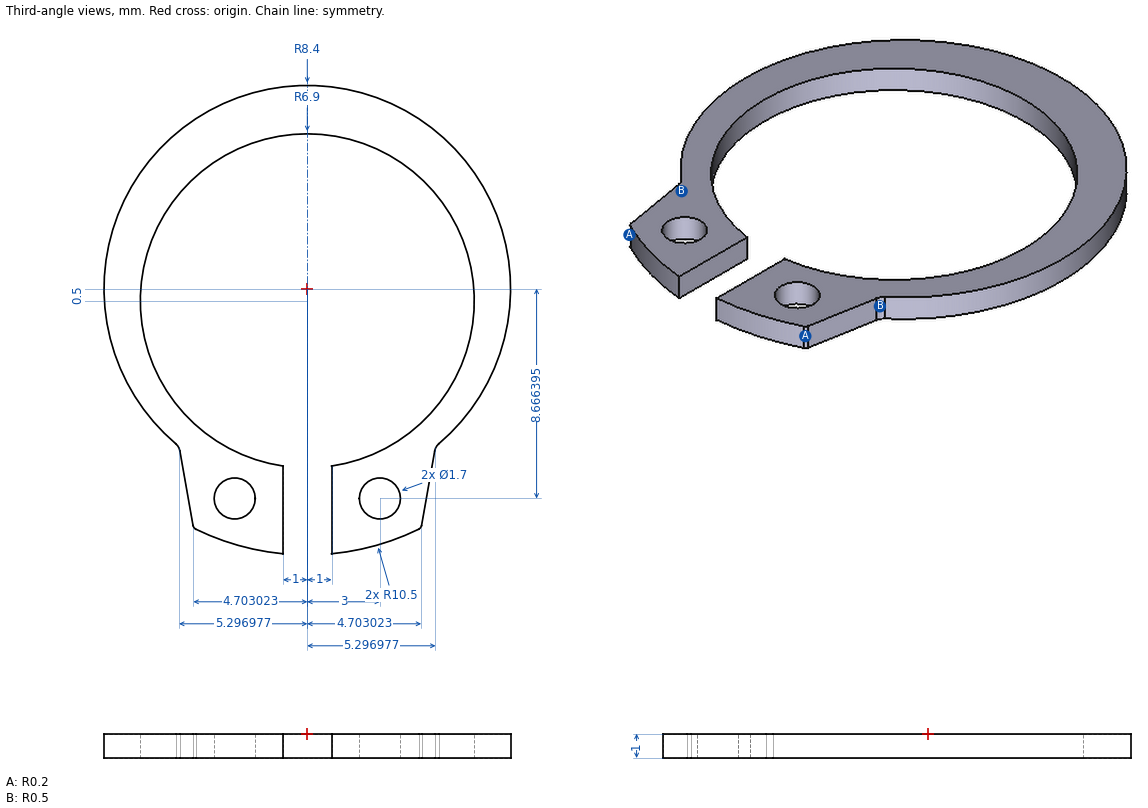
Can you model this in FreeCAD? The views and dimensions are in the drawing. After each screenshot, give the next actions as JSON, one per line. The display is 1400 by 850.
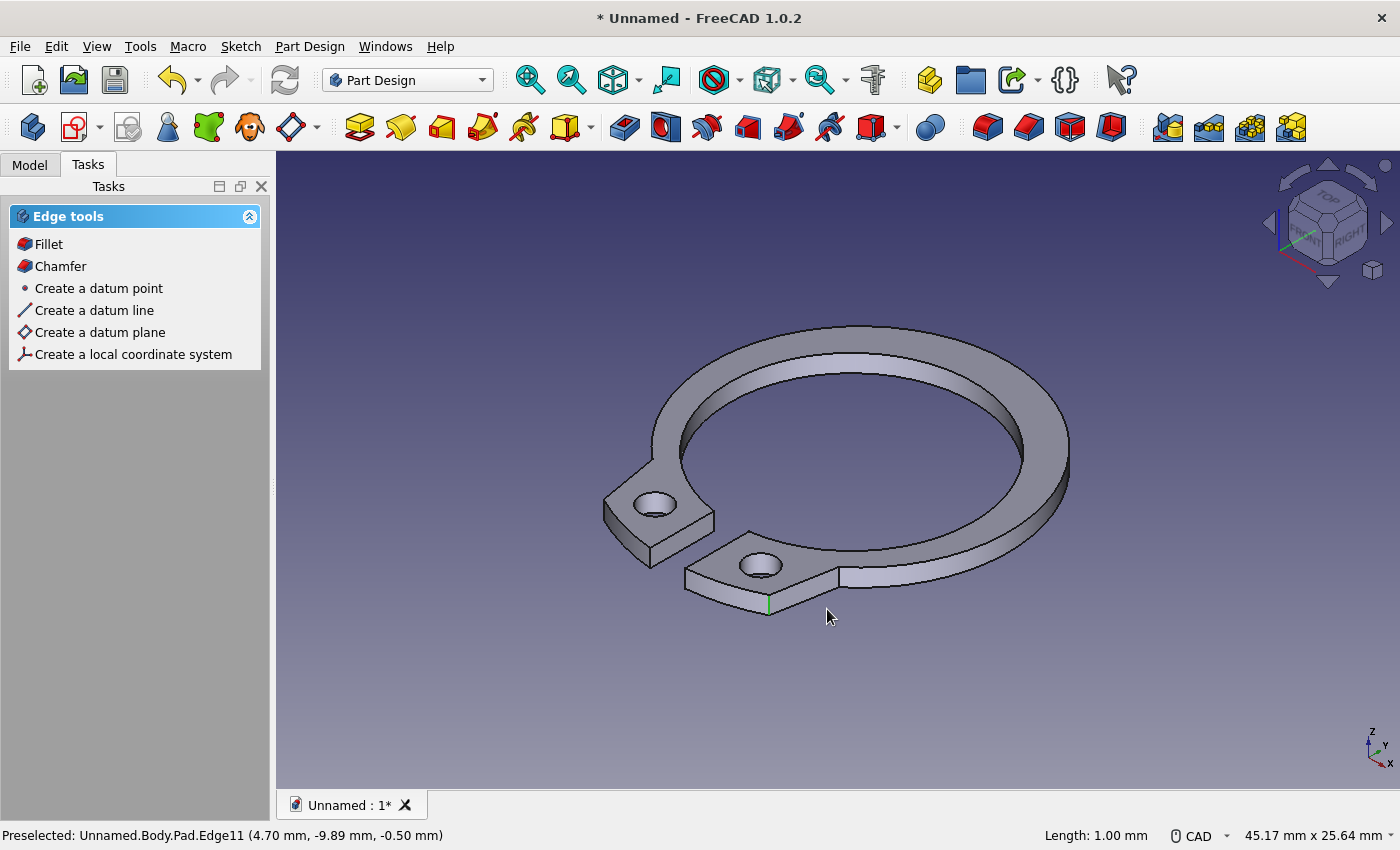
{"action": "key", "text": "2"}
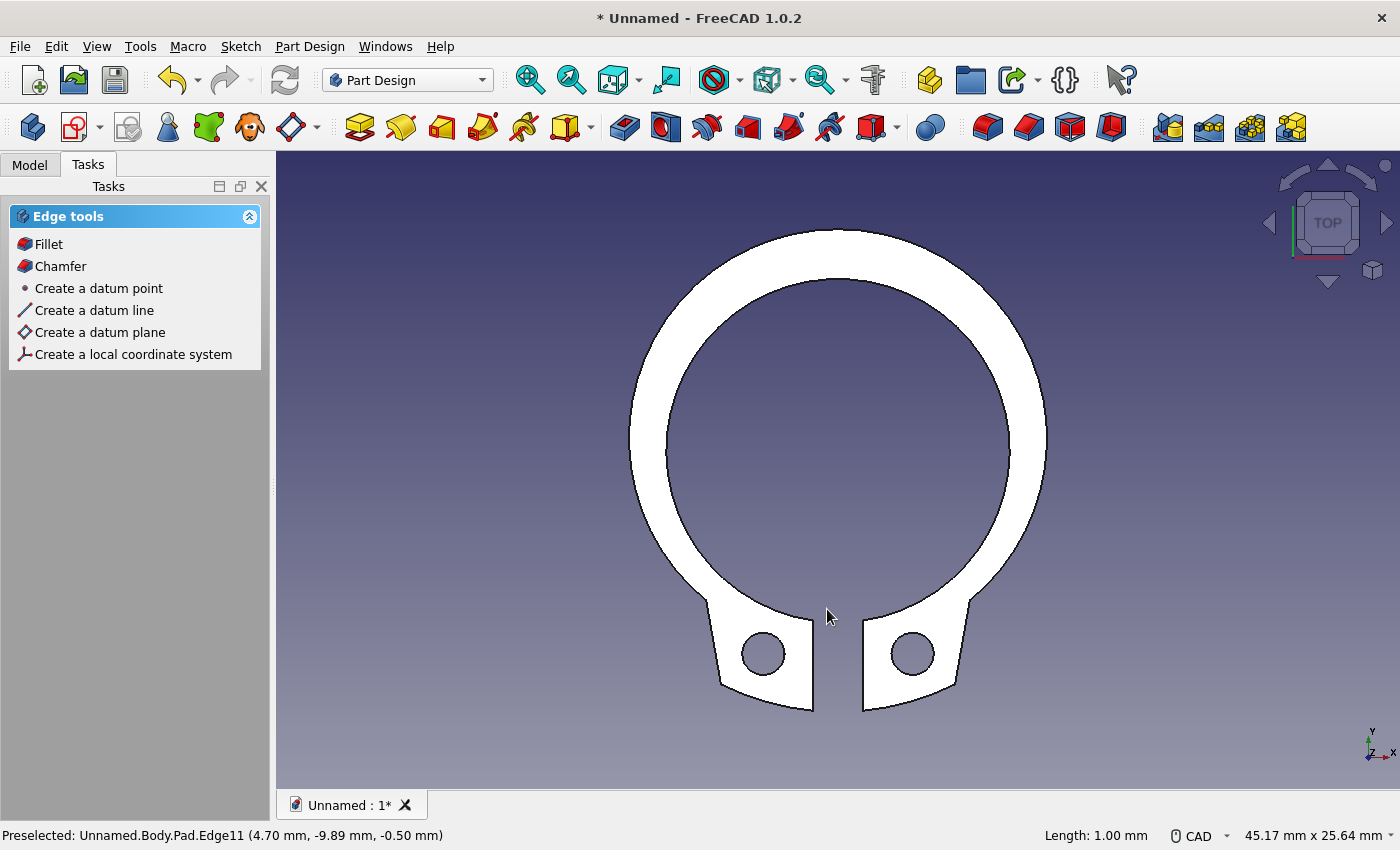
{"action": "key", "text": "1"}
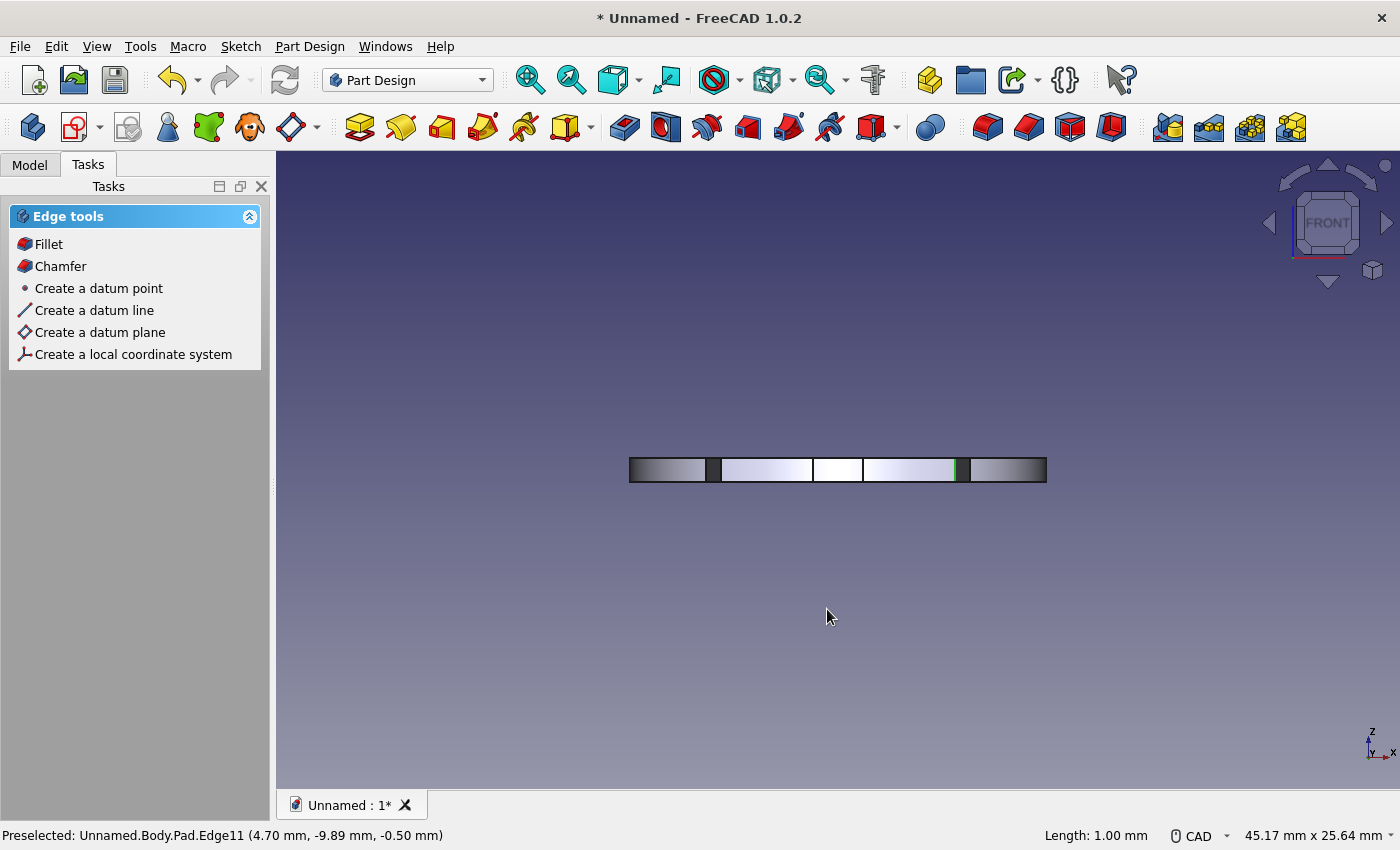
{"action": "left_click", "coordinate": [531, 80]}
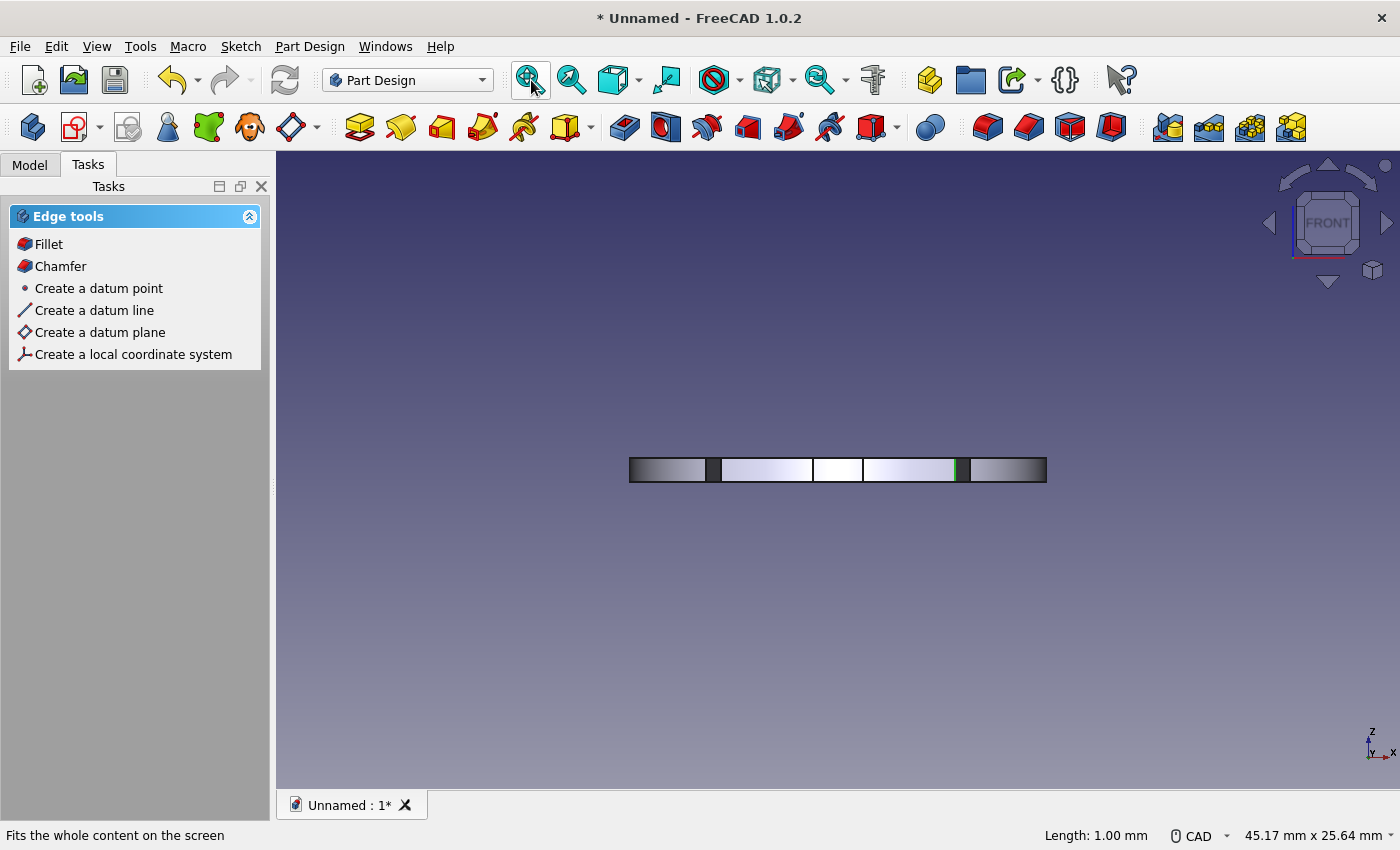
{"action": "key", "text": "3"}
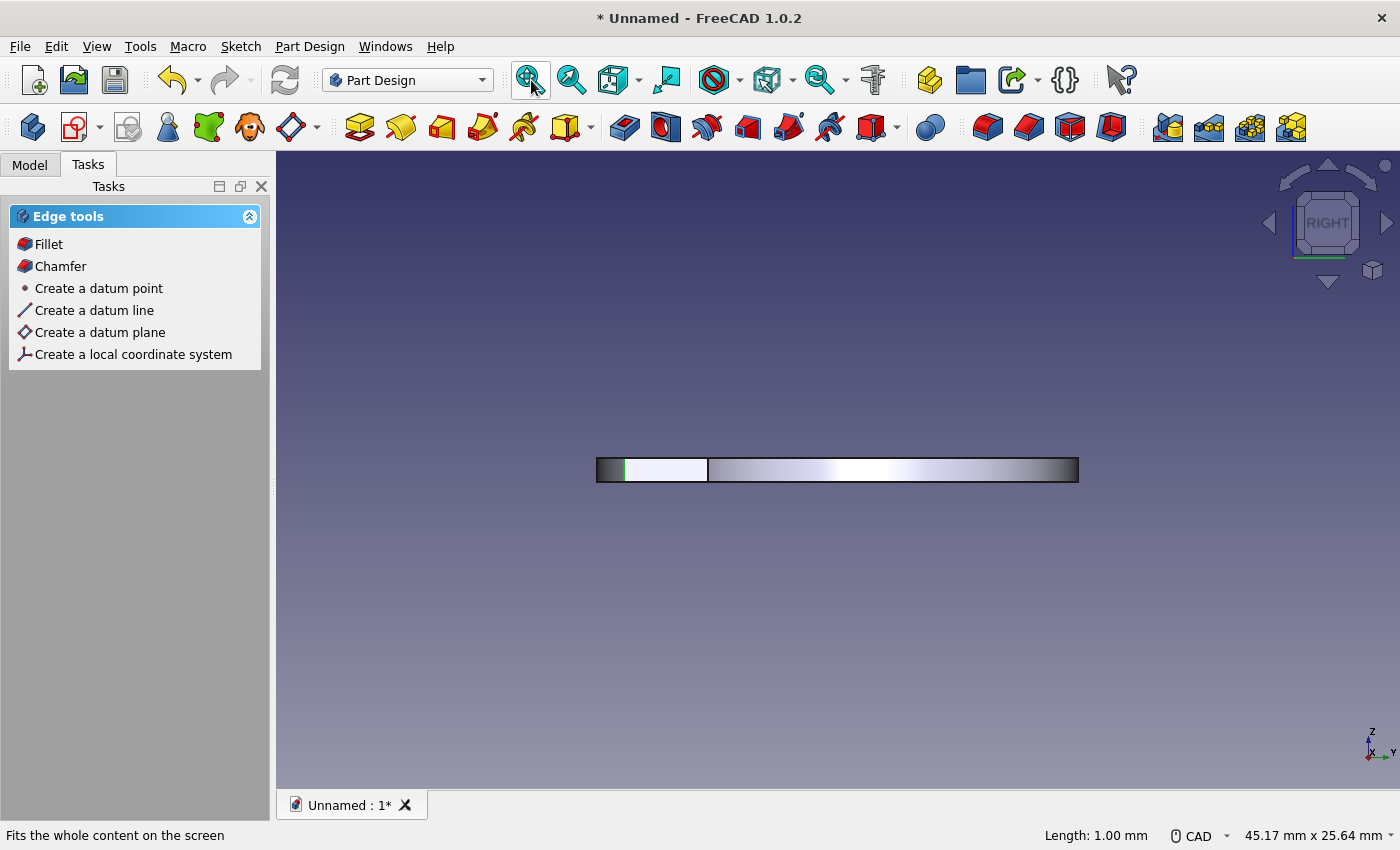
{"action": "left_click", "coordinate": [531, 80]}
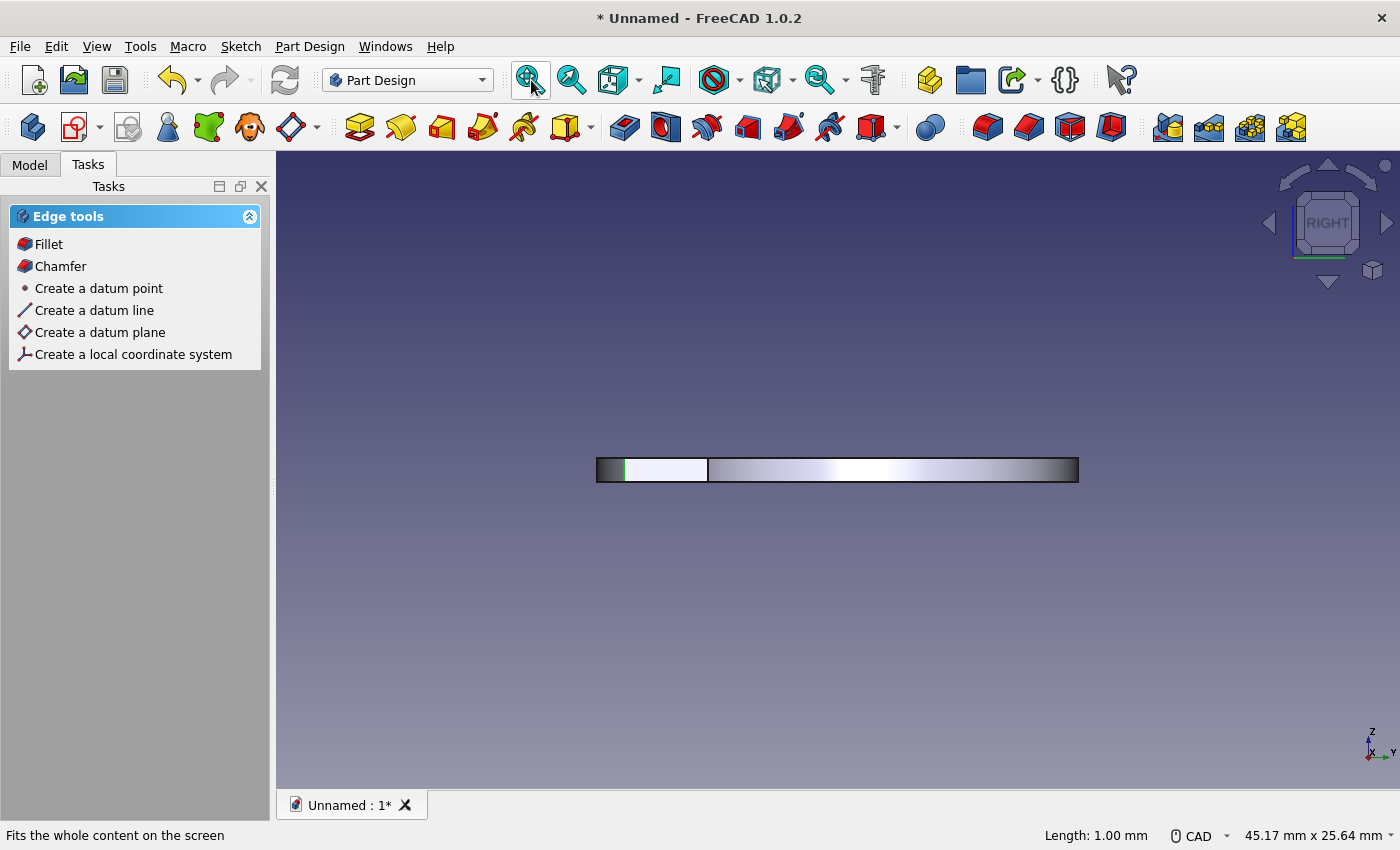
{"action": "key", "text": "5"}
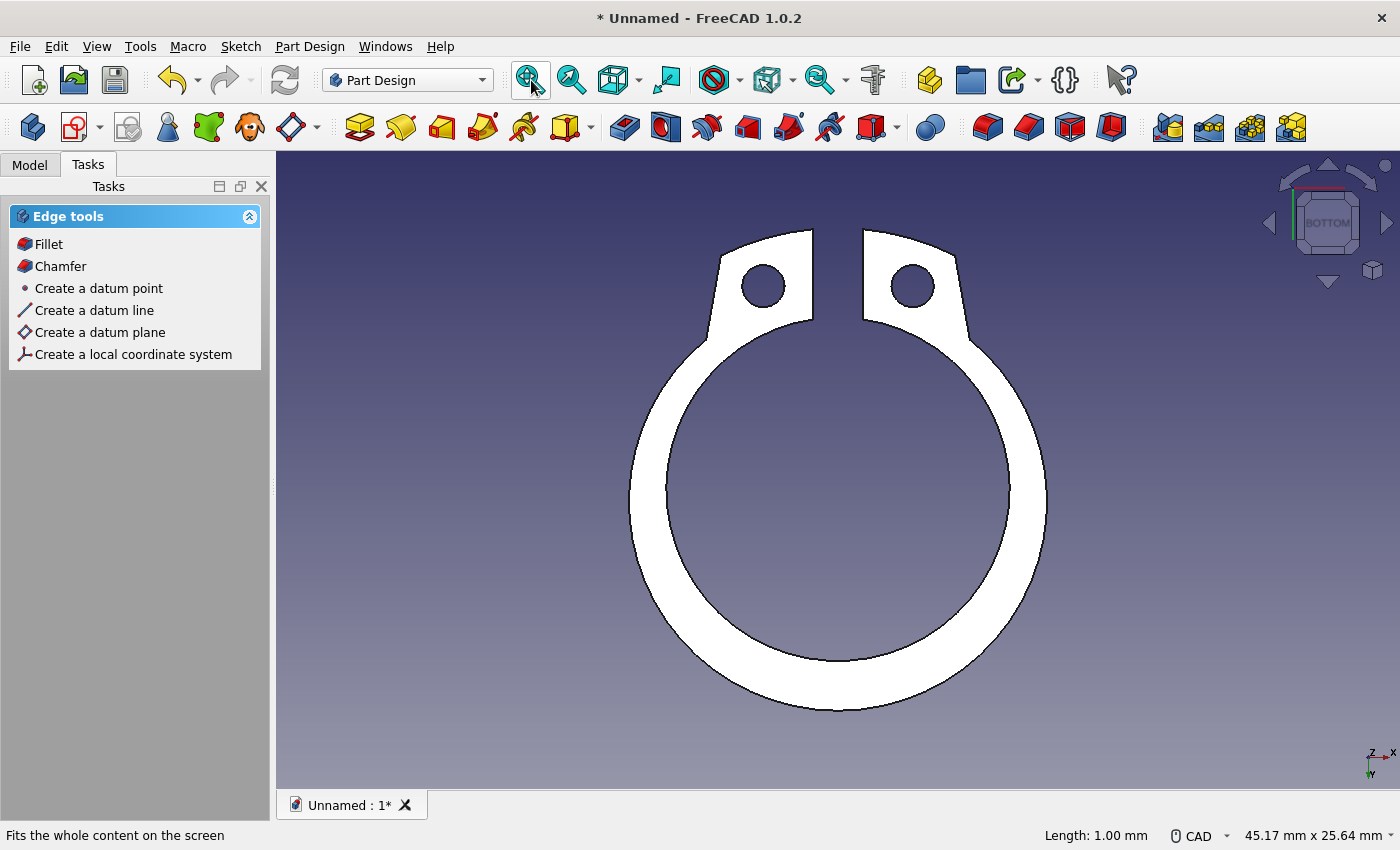
{"action": "key", "text": "4"}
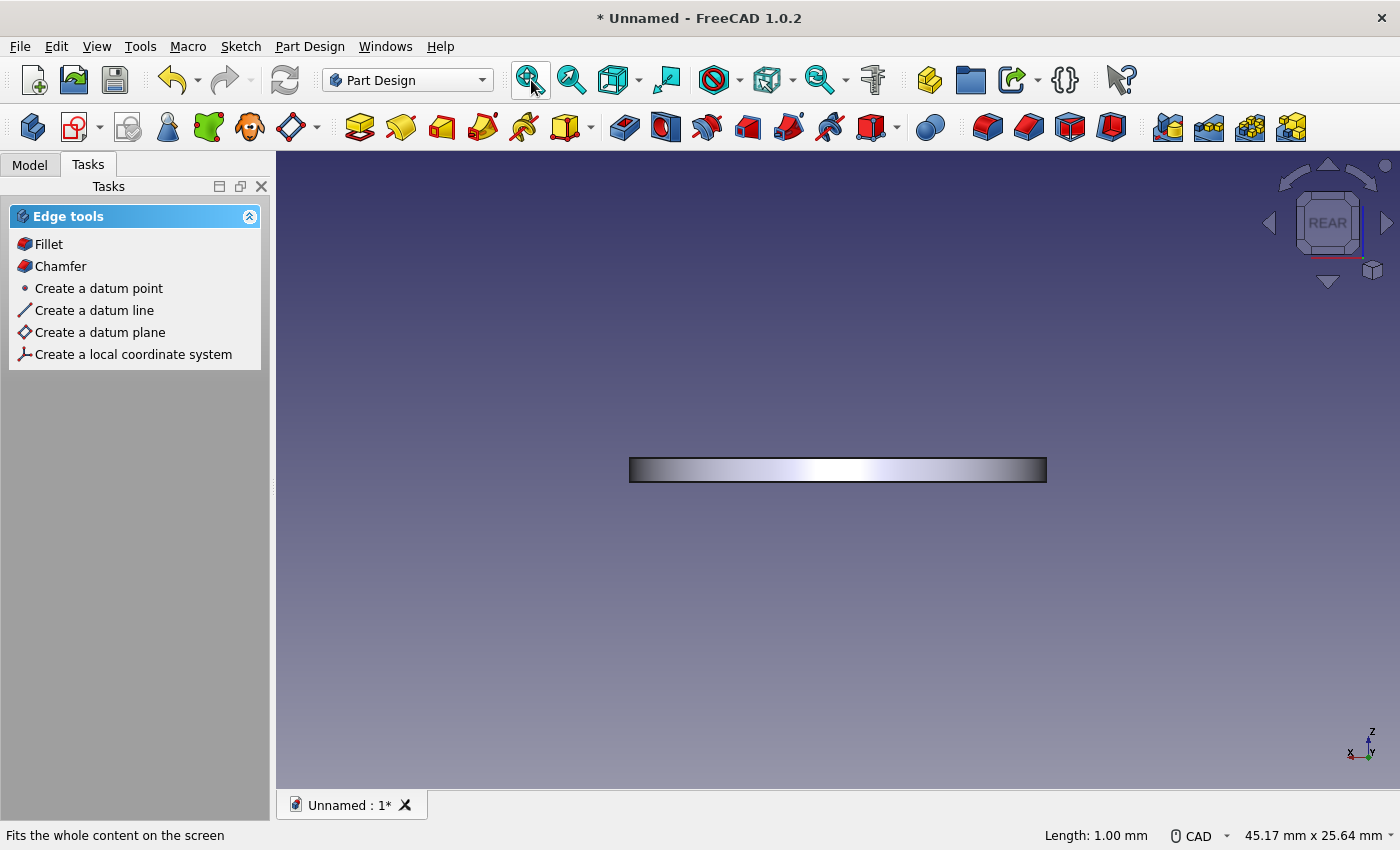
{"action": "left_click", "coordinate": [531, 80]}